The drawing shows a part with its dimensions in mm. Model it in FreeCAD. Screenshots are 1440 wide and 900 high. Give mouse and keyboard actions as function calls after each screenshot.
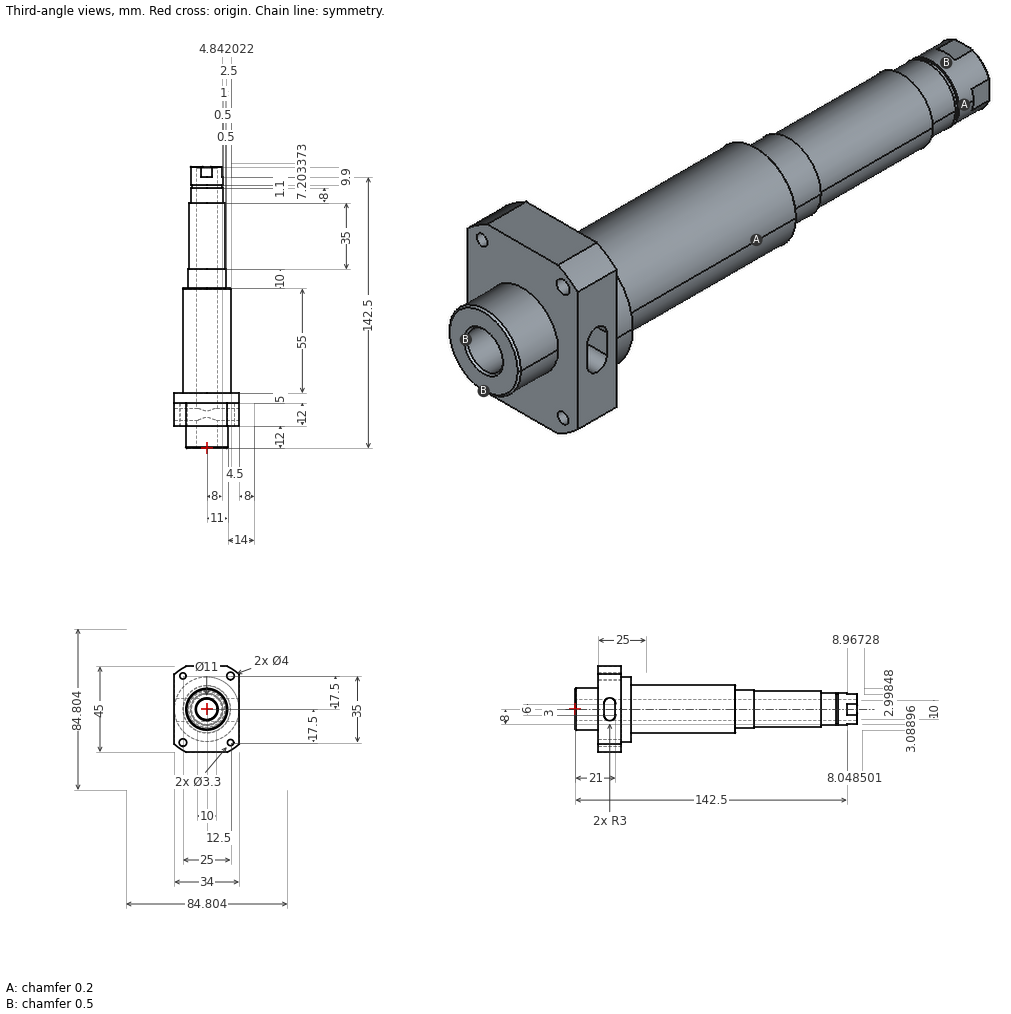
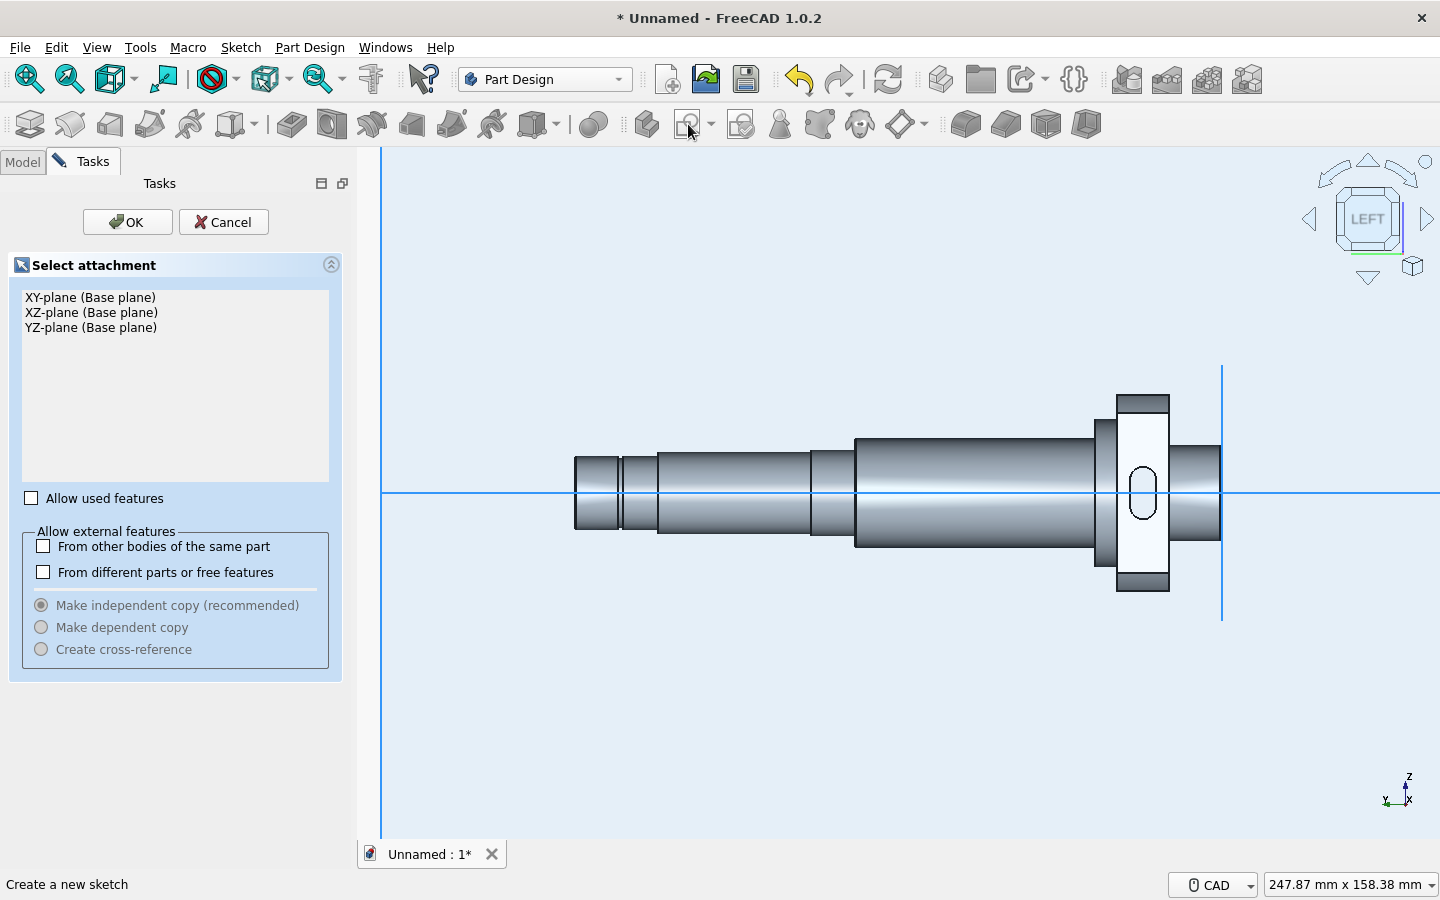
click(82, 328)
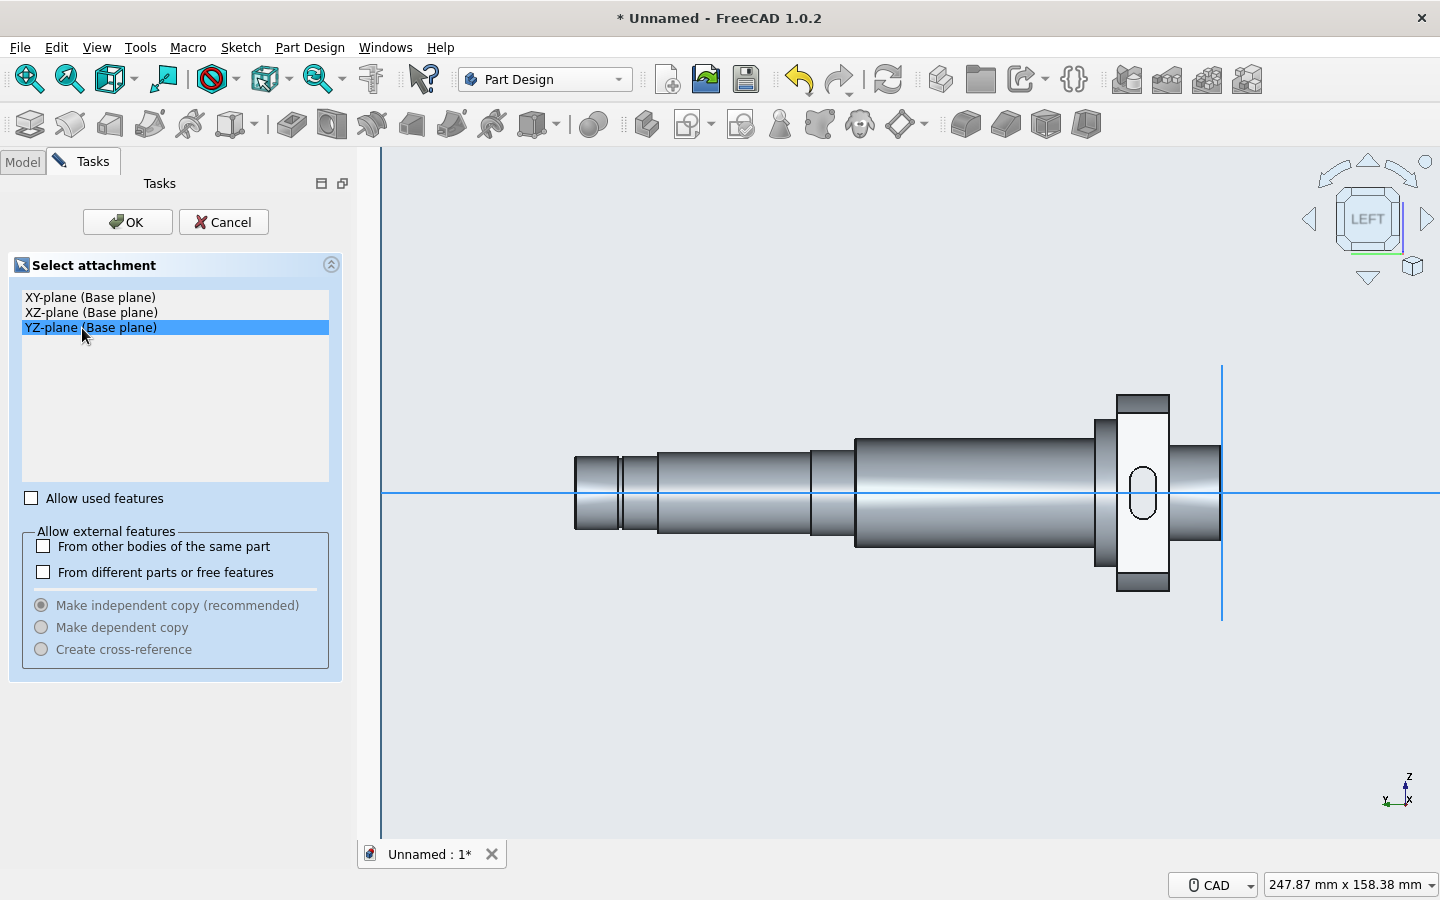
click(128, 222)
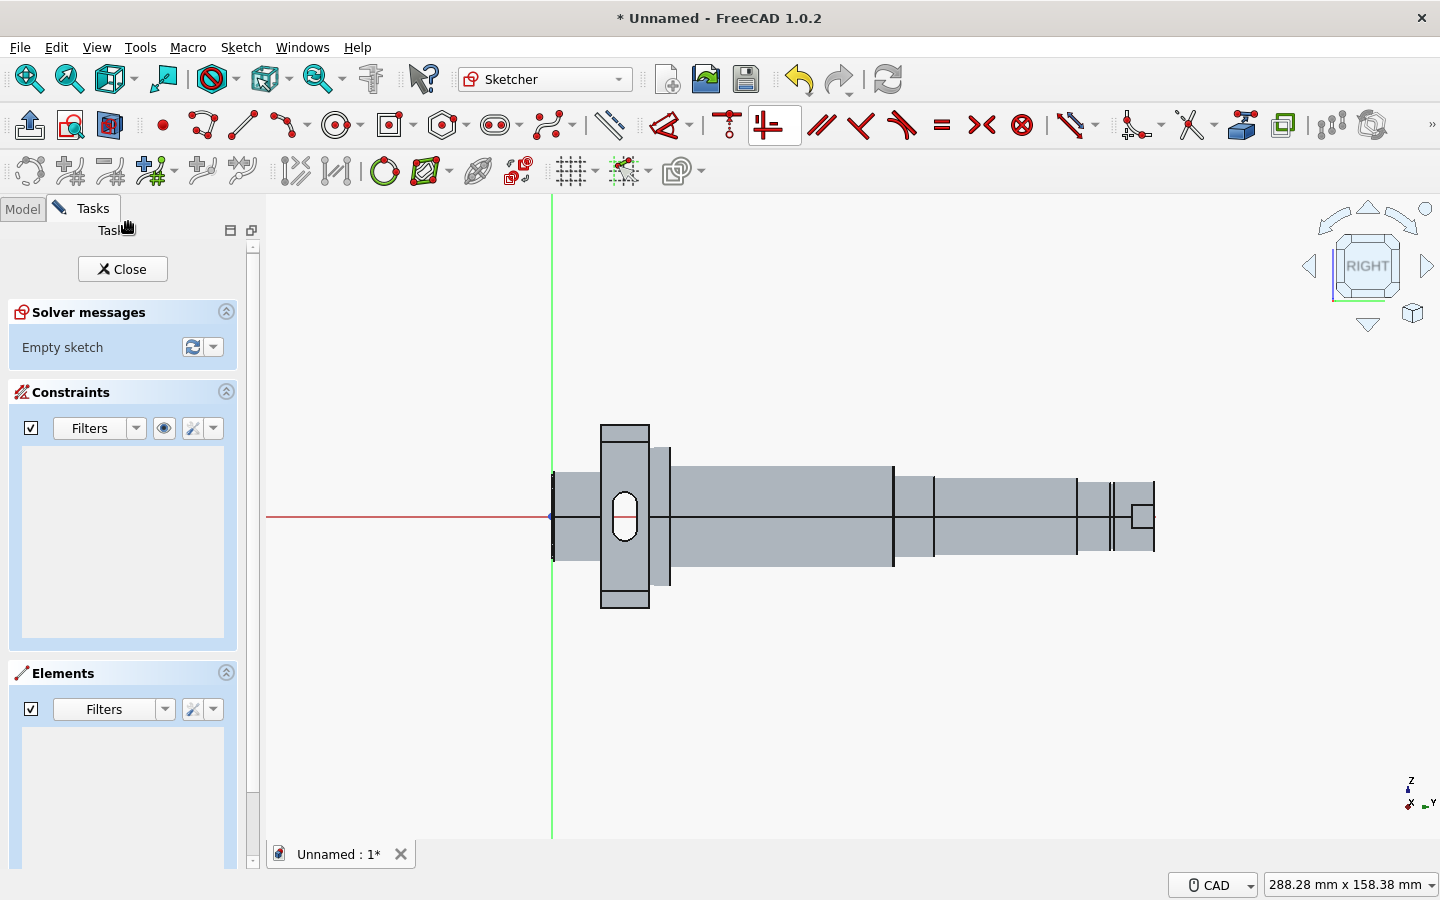
click(110, 126)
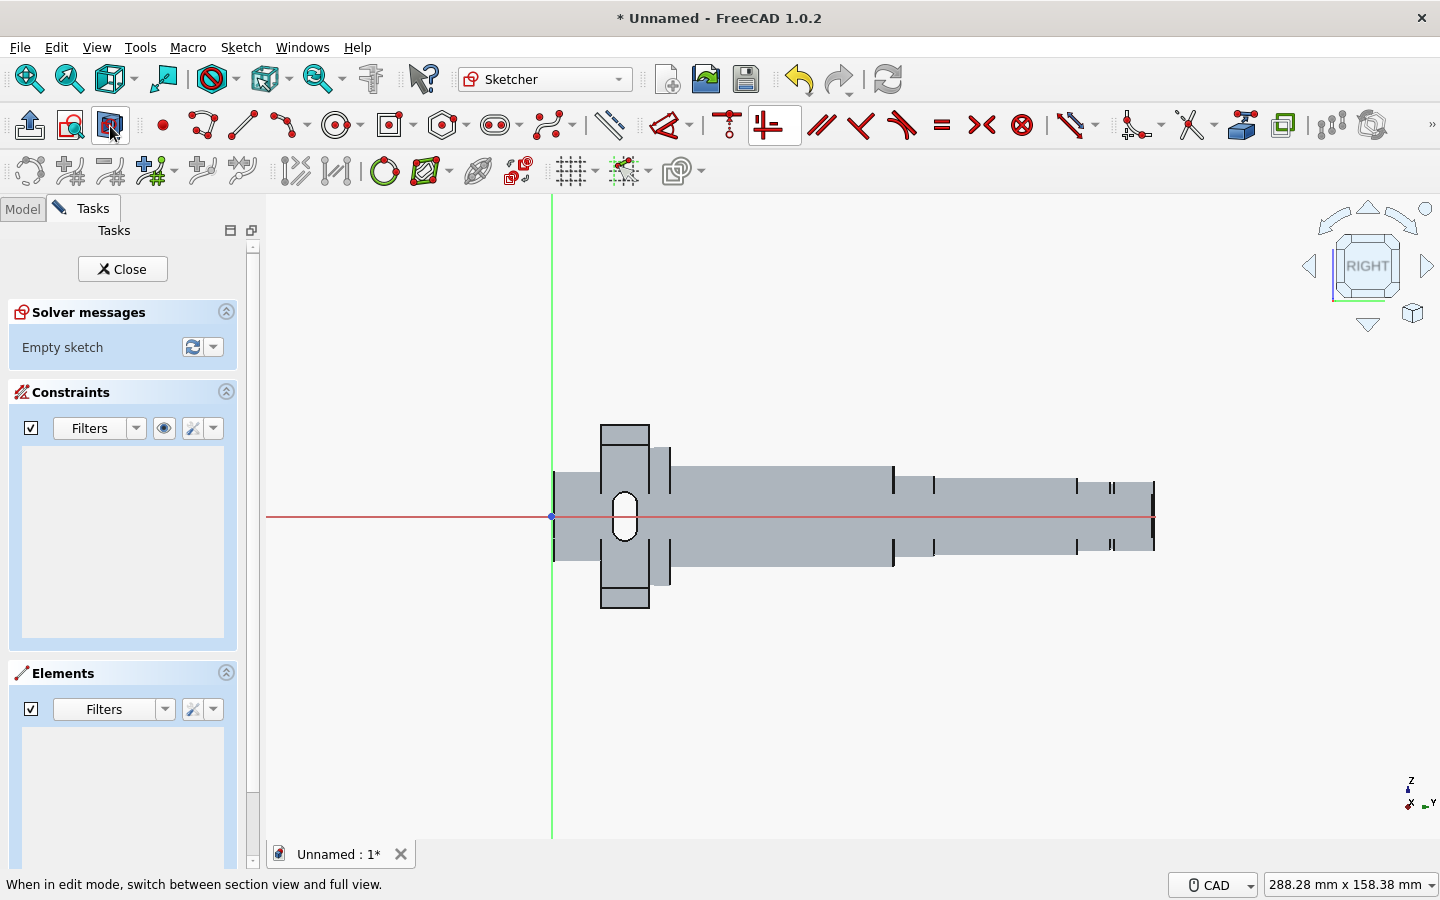
scroll(1243, 517, up, 8)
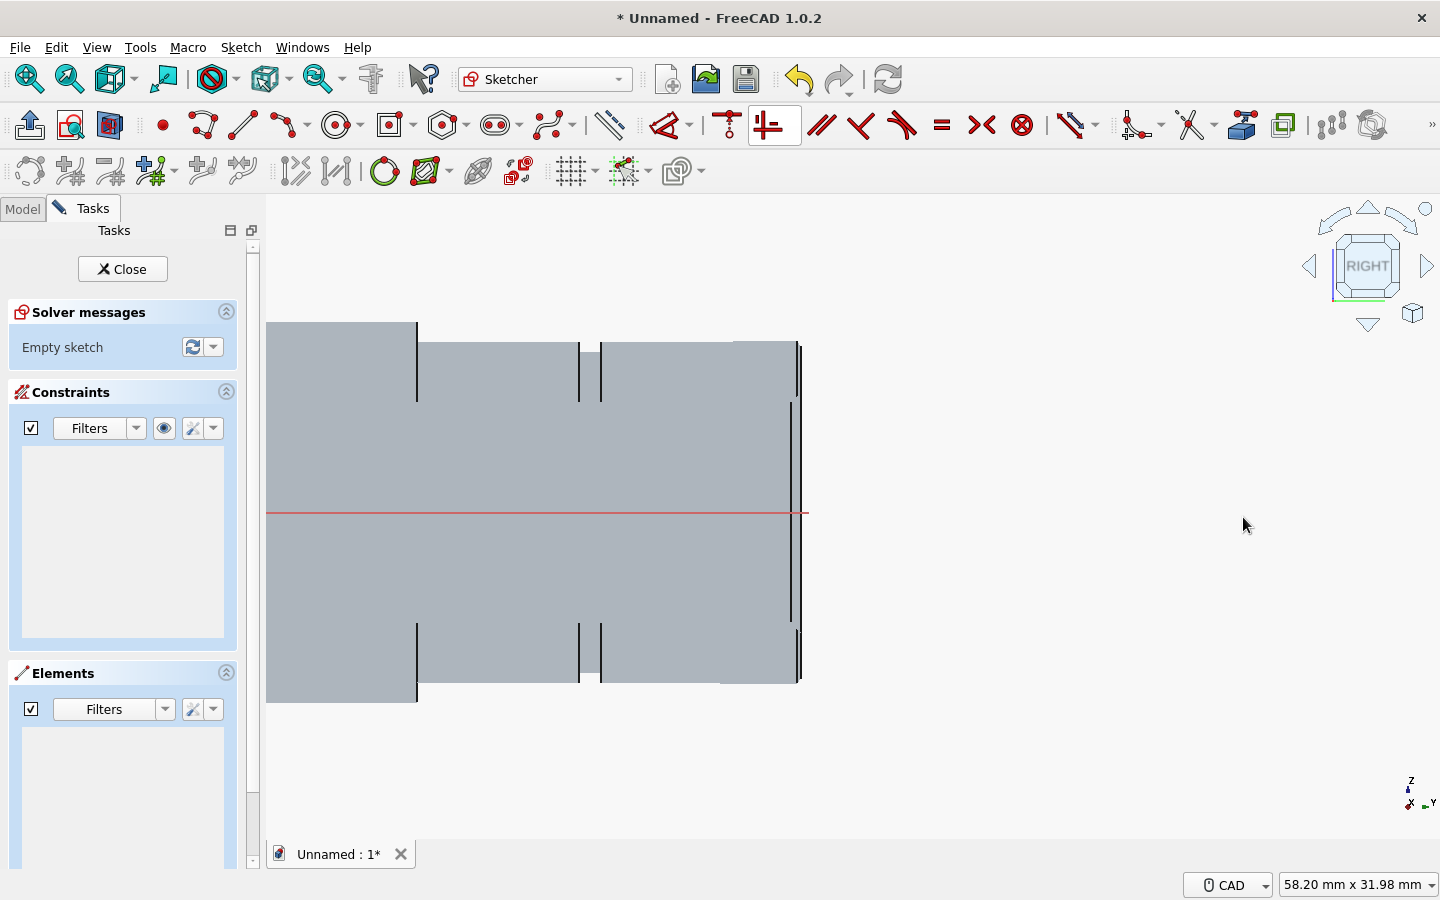
key(g)
key(r)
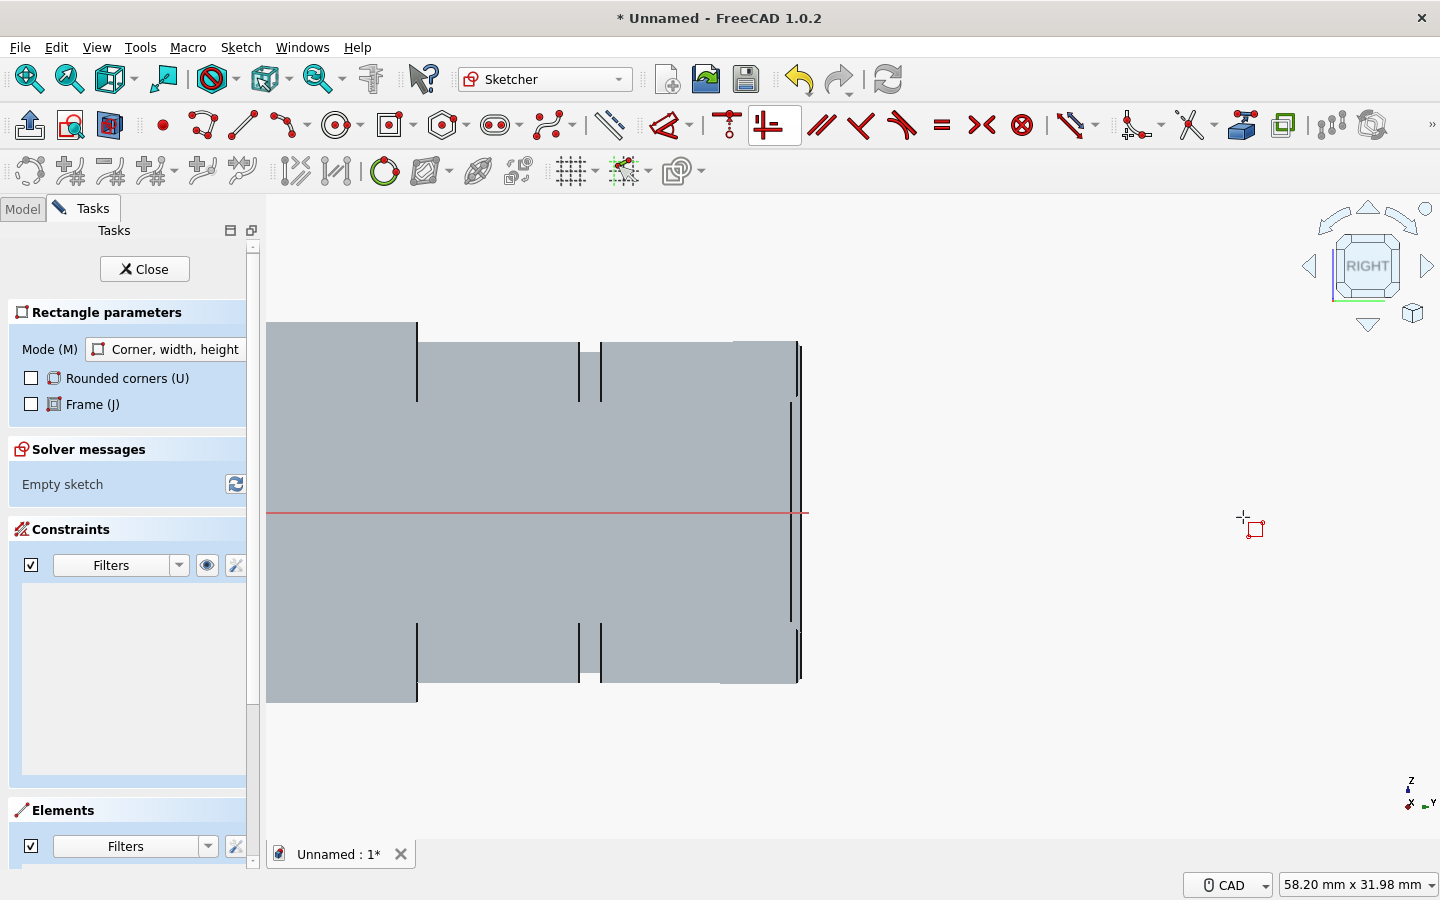
click(690, 674)
move(852, 736)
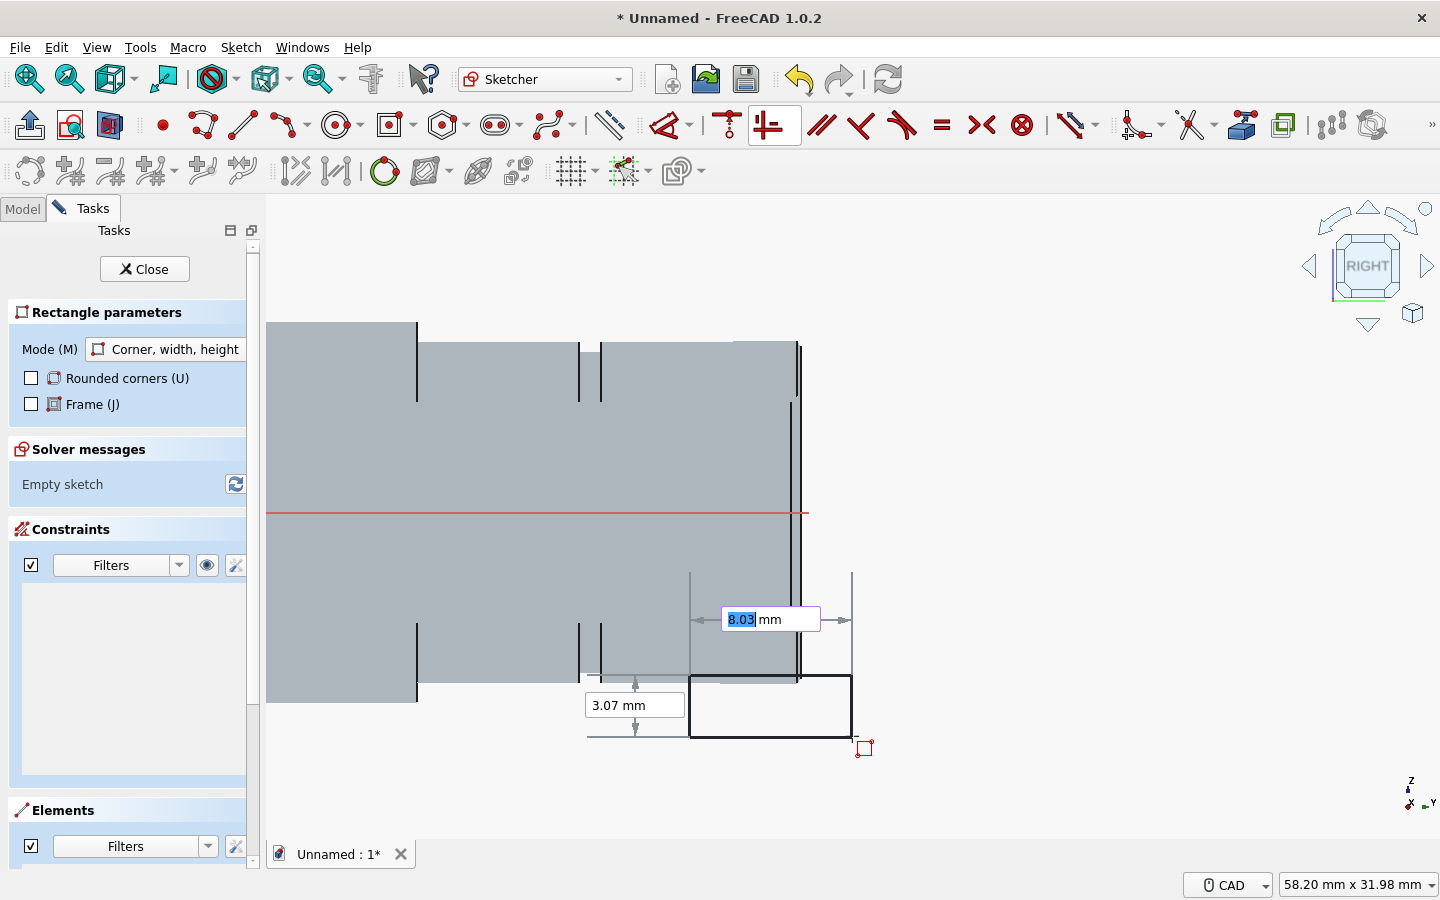
text(8.048501)
key(Tab)
text(3.08896)
key(Return)